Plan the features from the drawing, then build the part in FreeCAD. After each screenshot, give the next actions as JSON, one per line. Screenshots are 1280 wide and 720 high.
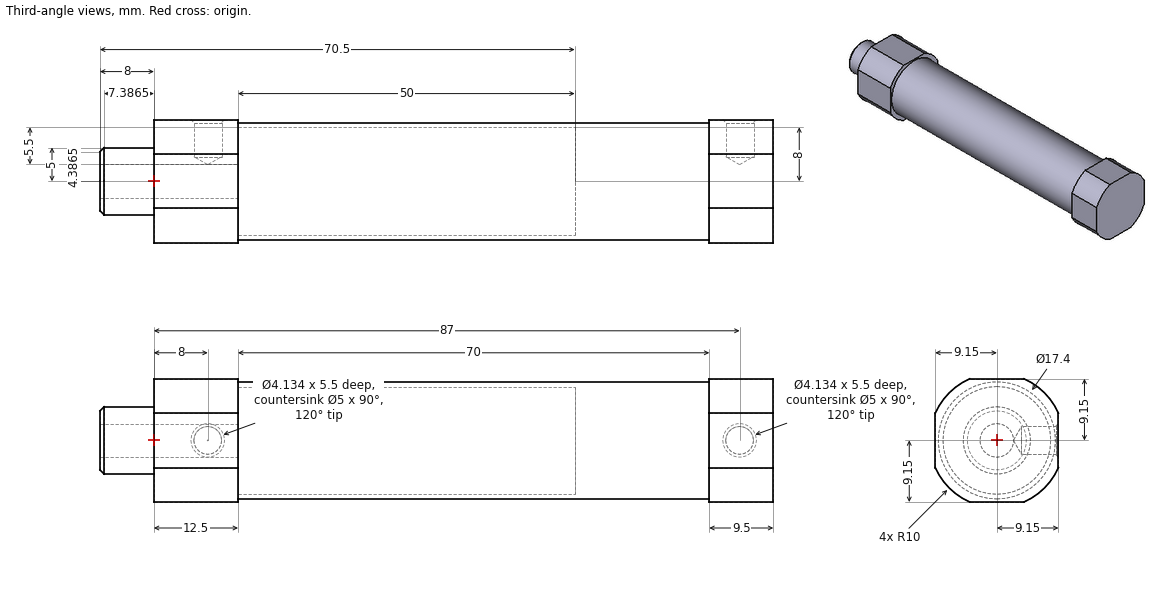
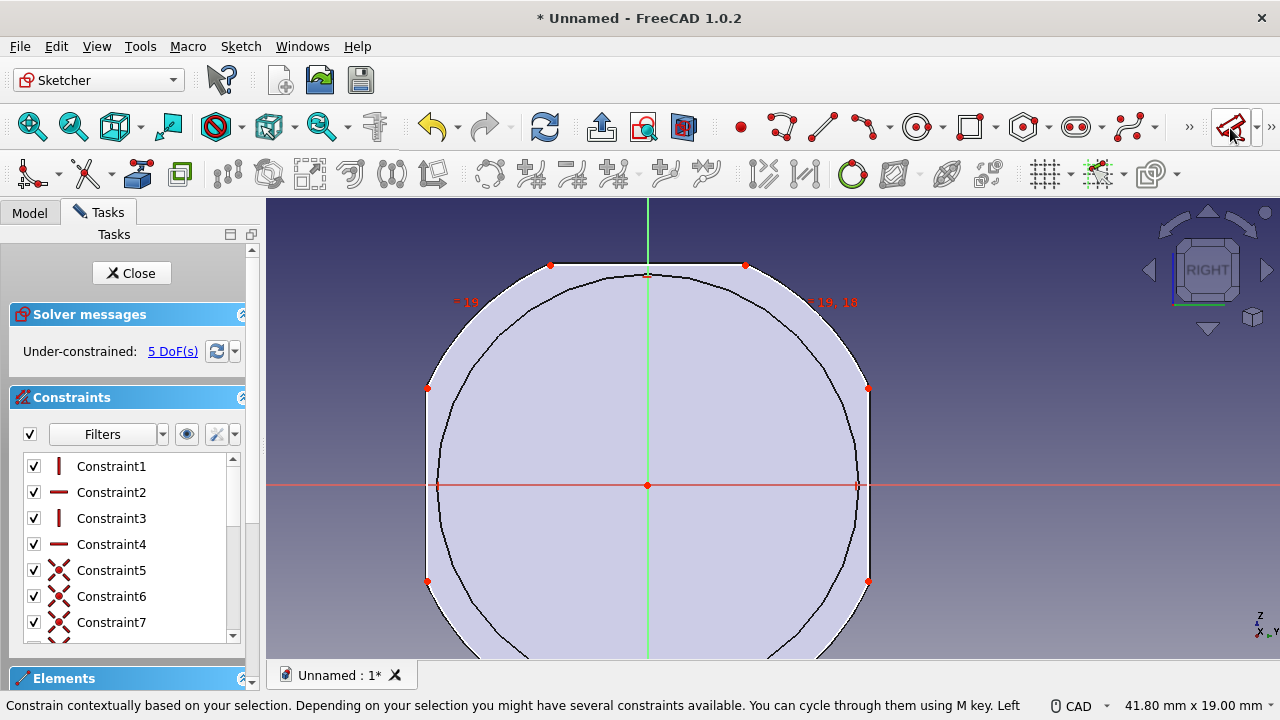
{"action": "left_click", "coordinate": [454, 628]}
{"action": "left_click", "coordinate": [378, 522]}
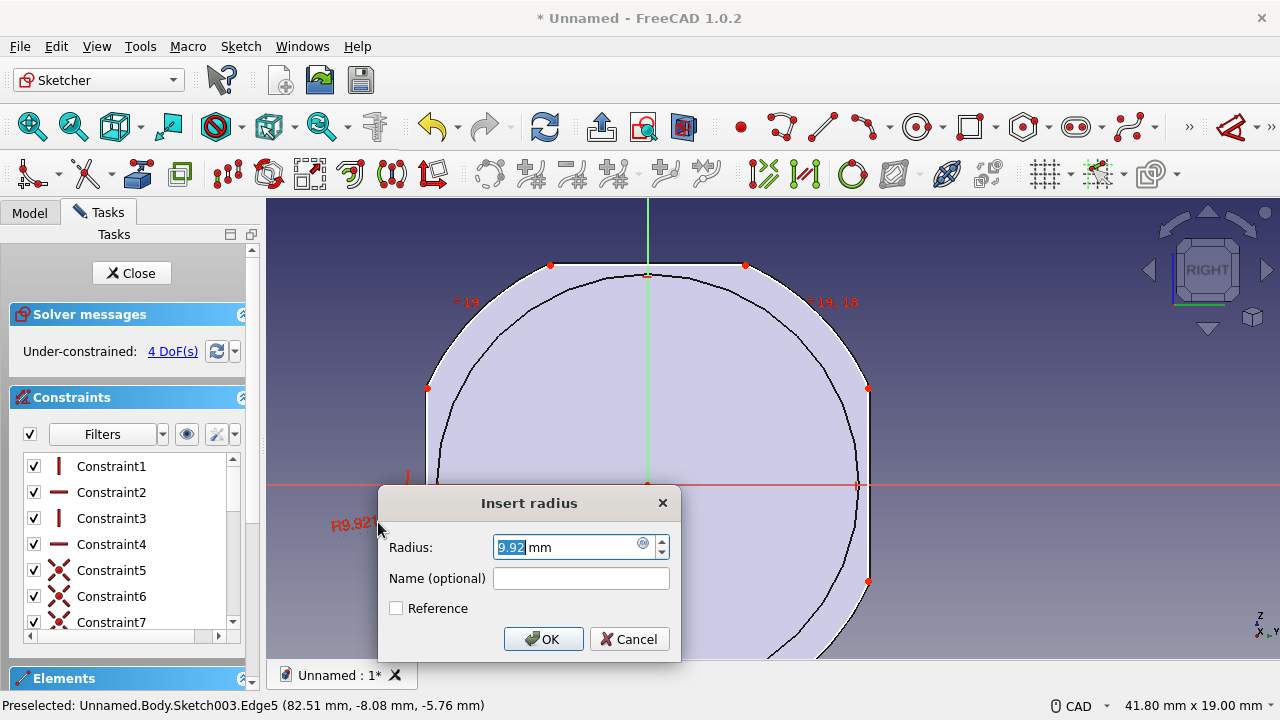
{"action": "type", "text": "10"}
{"action": "key", "text": "Return"}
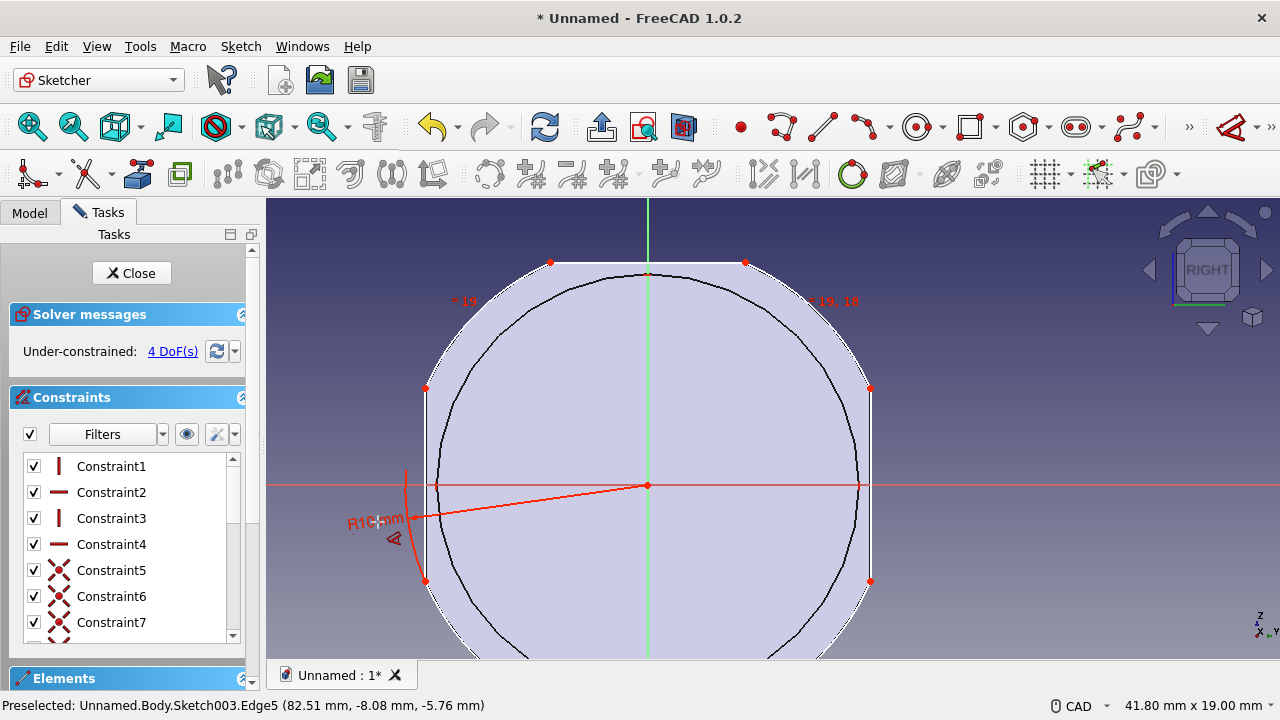
{"action": "left_click", "coordinate": [425, 389]}
{"action": "left_click", "coordinate": [537, 355]}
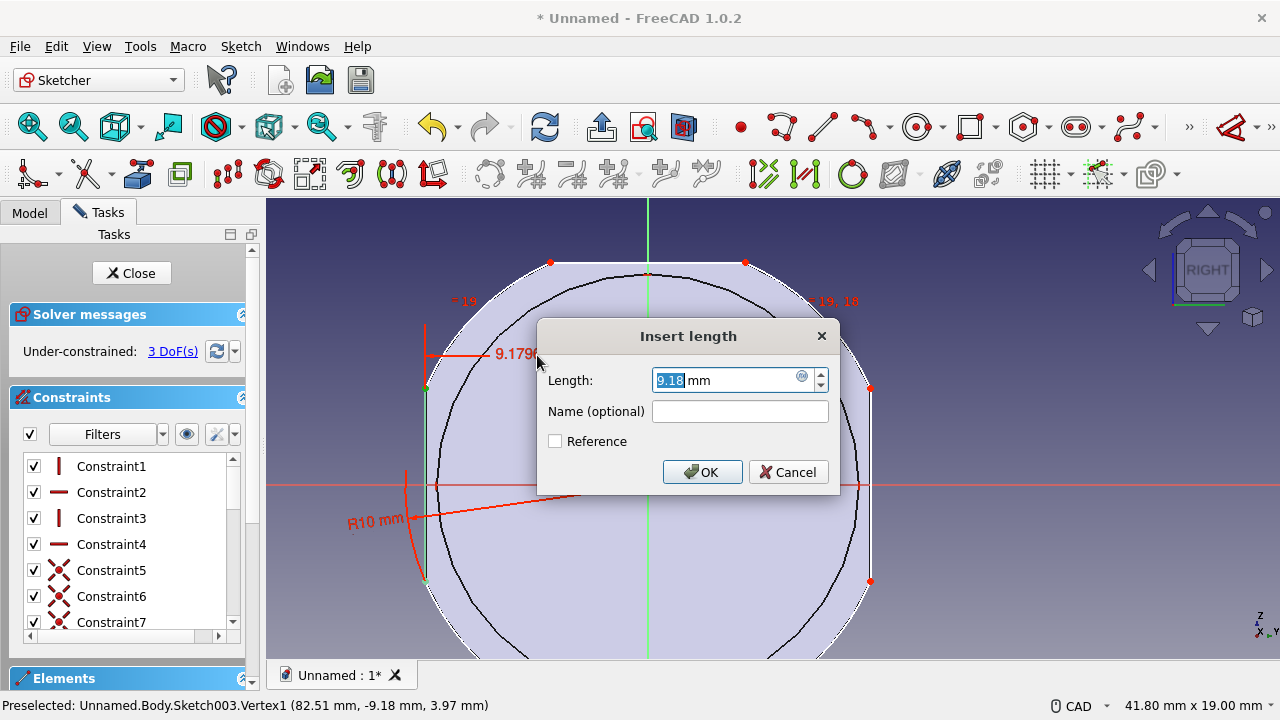
{"action": "type", "text": "9.15"}
{"action": "key", "text": "Return"}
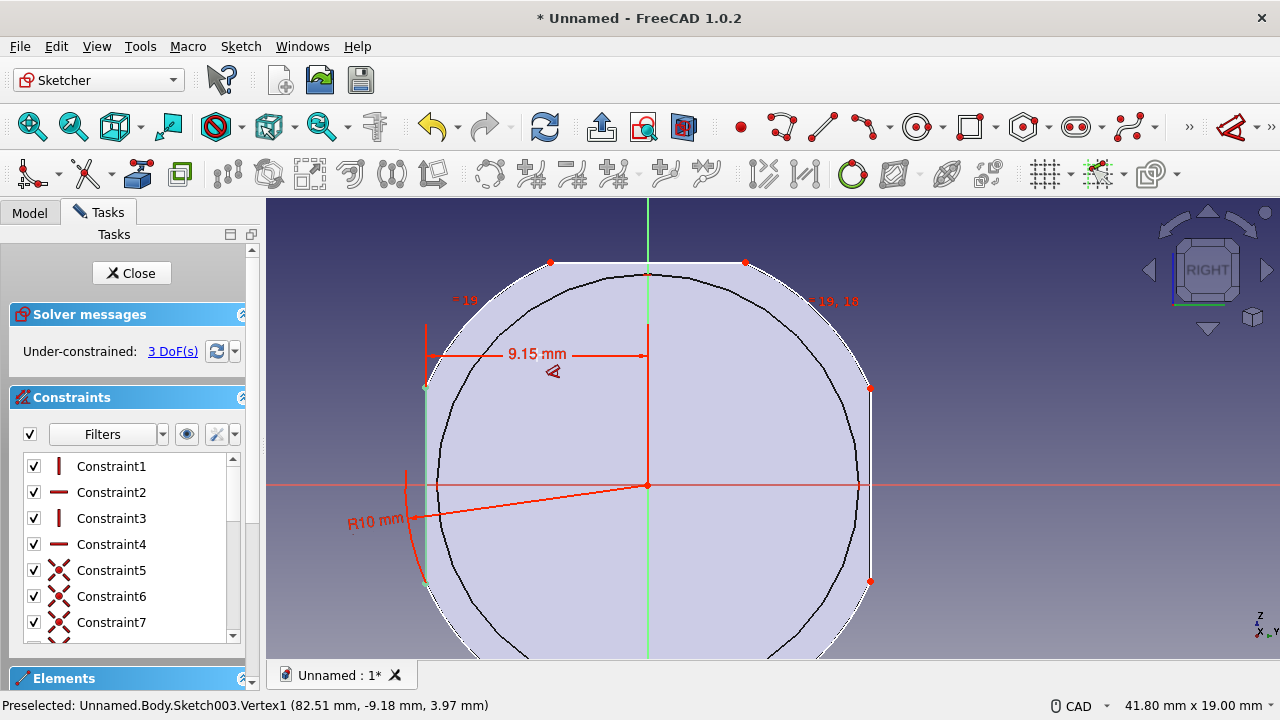
{"action": "scroll", "coordinate": [820, 313], "scroll_direction": "down", "scroll_amount": 2}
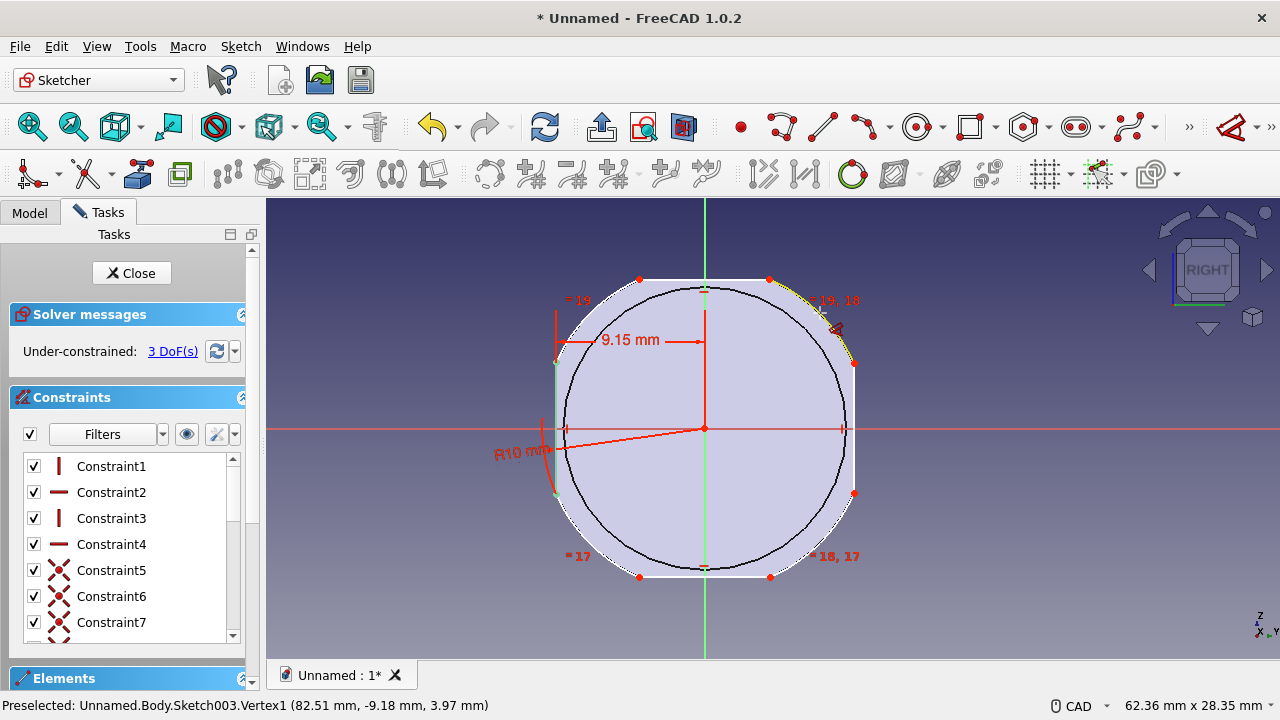
{"action": "left_click", "coordinate": [640, 577]}
{"action": "left_click", "coordinate": [606, 503]}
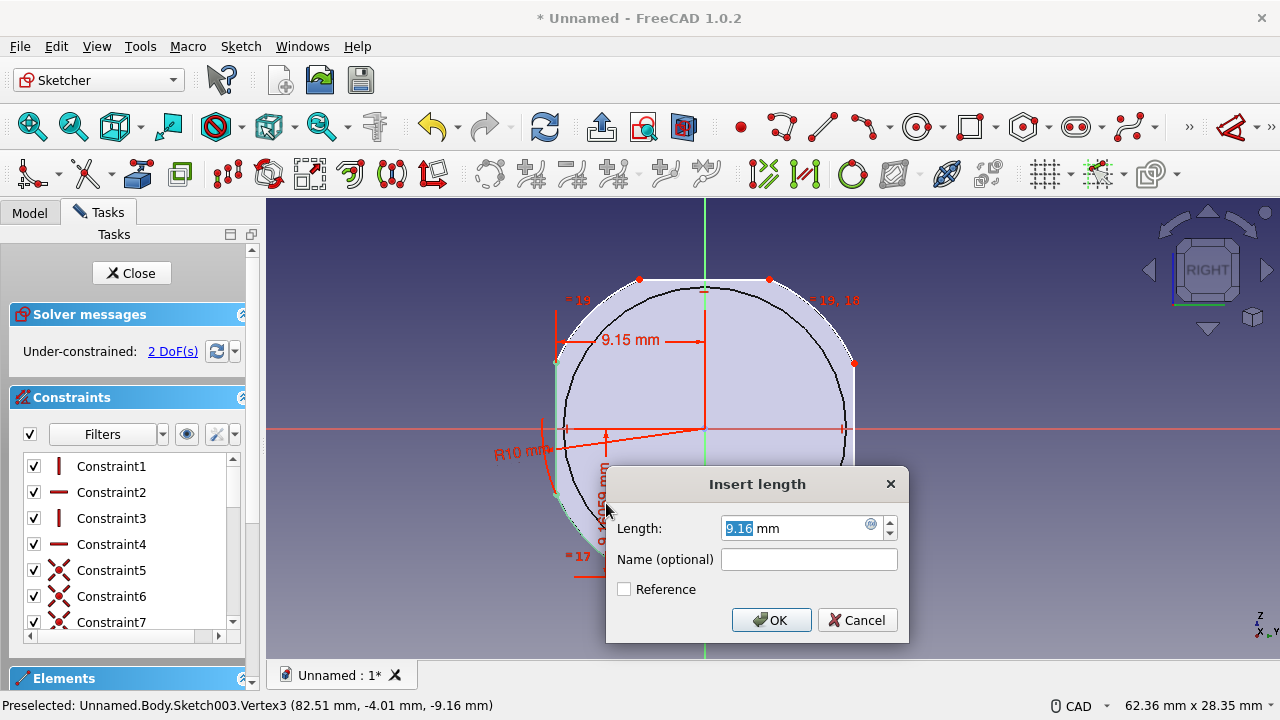
{"action": "type", "text": "9.15"}
{"action": "key", "text": "Return"}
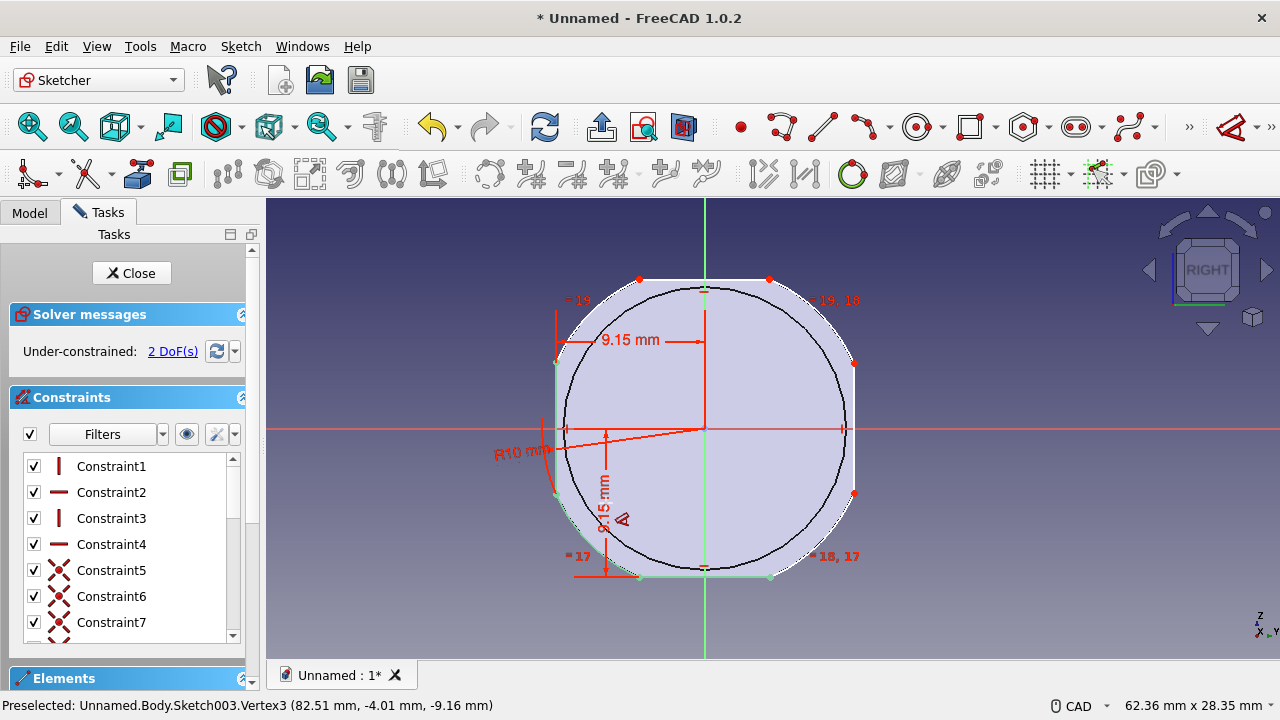
{"action": "left_click", "coordinate": [854, 493]}
{"action": "left_click", "coordinate": [779, 527]}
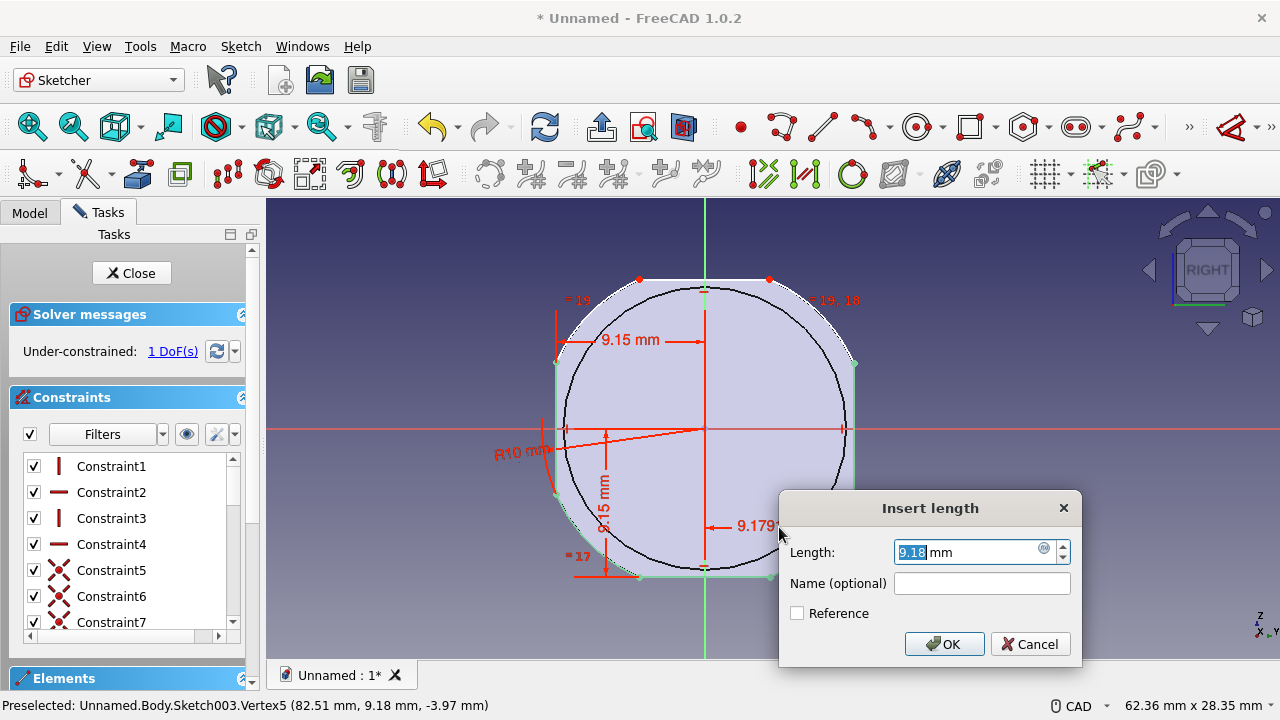
{"action": "type", "text": "9.15"}
{"action": "key", "text": "Return"}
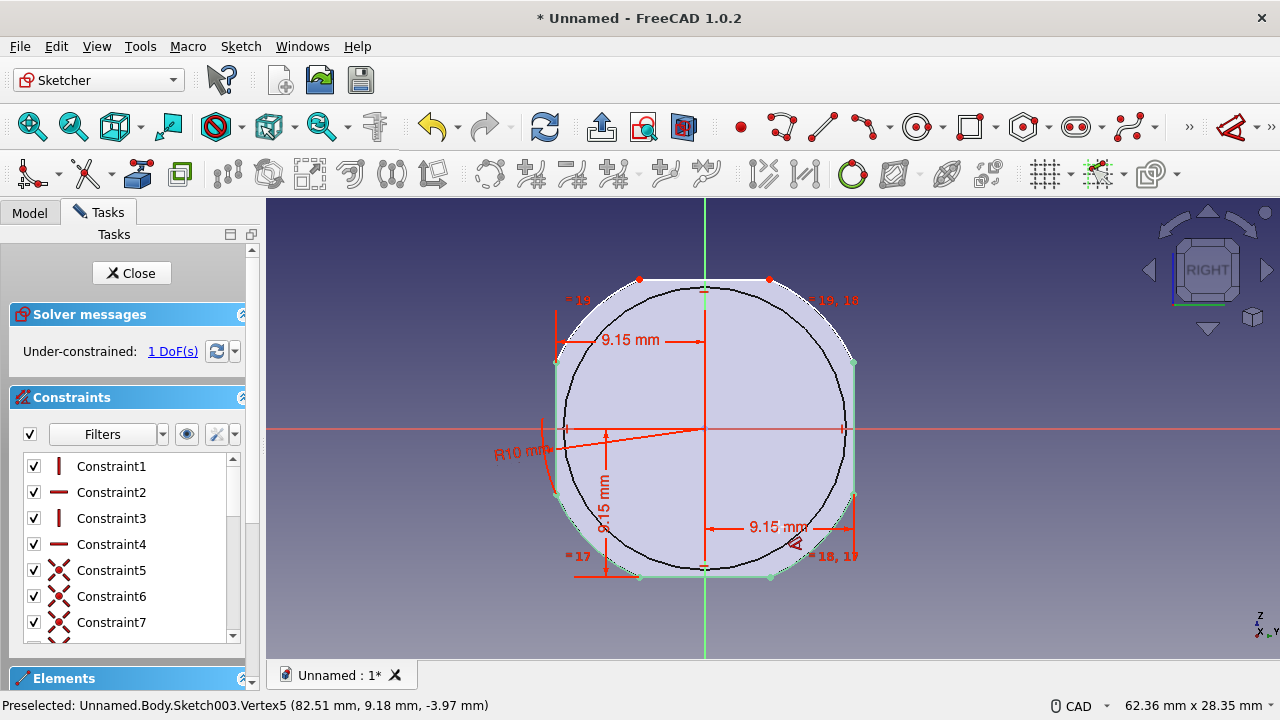
{"action": "left_click", "coordinate": [770, 280]}
{"action": "left_click", "coordinate": [804, 354]}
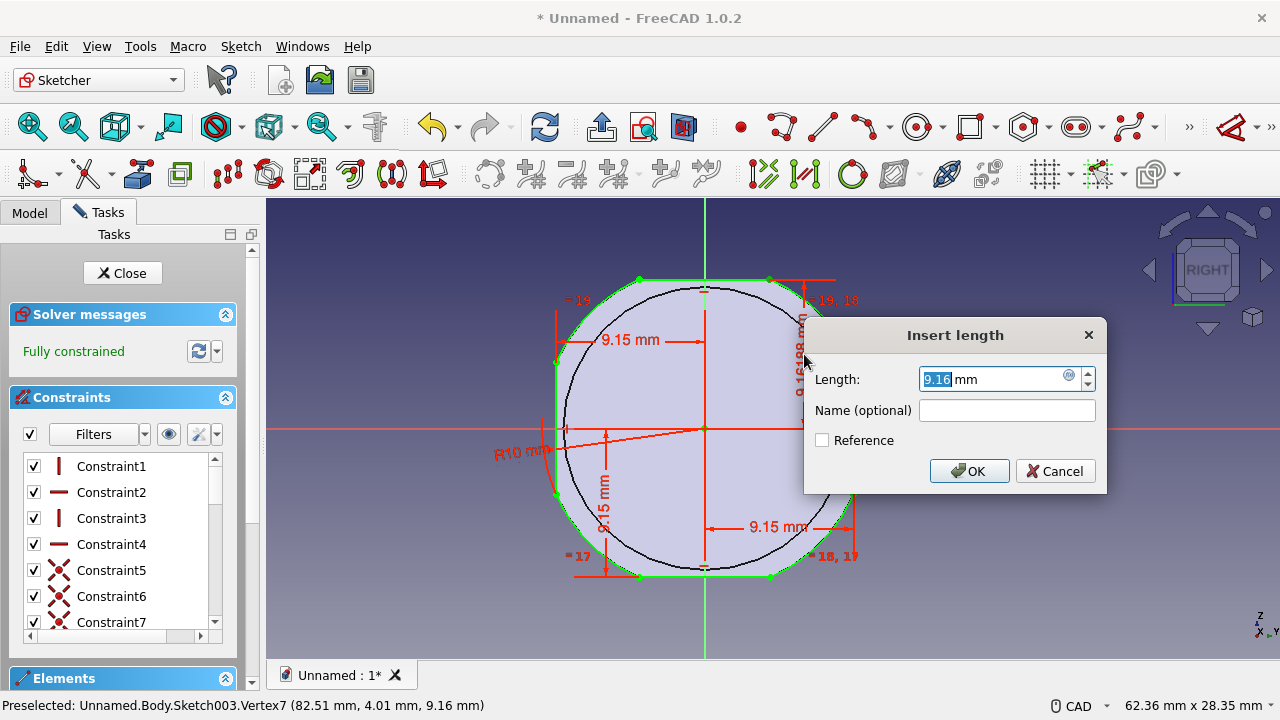
{"action": "type", "text": "9.15"}
{"action": "key", "text": "Return"}
{"action": "key", "text": "Escape"}